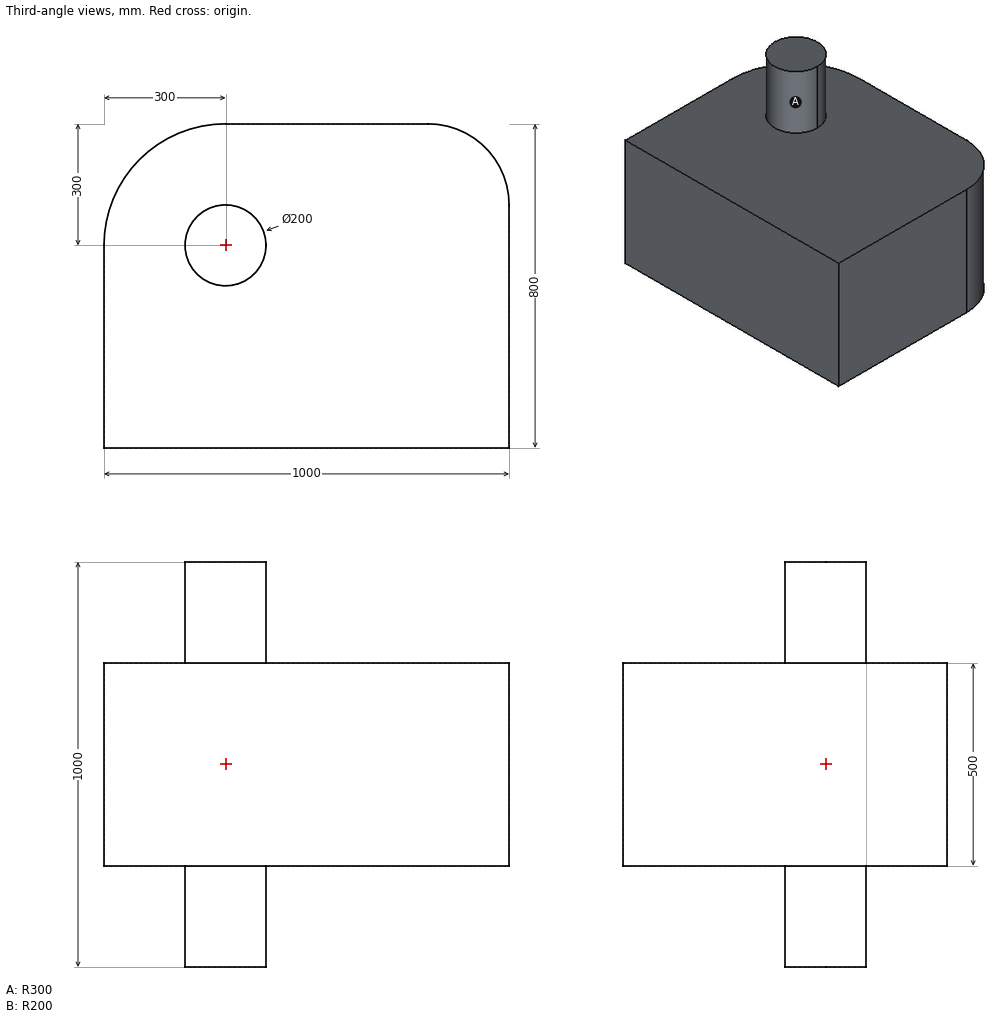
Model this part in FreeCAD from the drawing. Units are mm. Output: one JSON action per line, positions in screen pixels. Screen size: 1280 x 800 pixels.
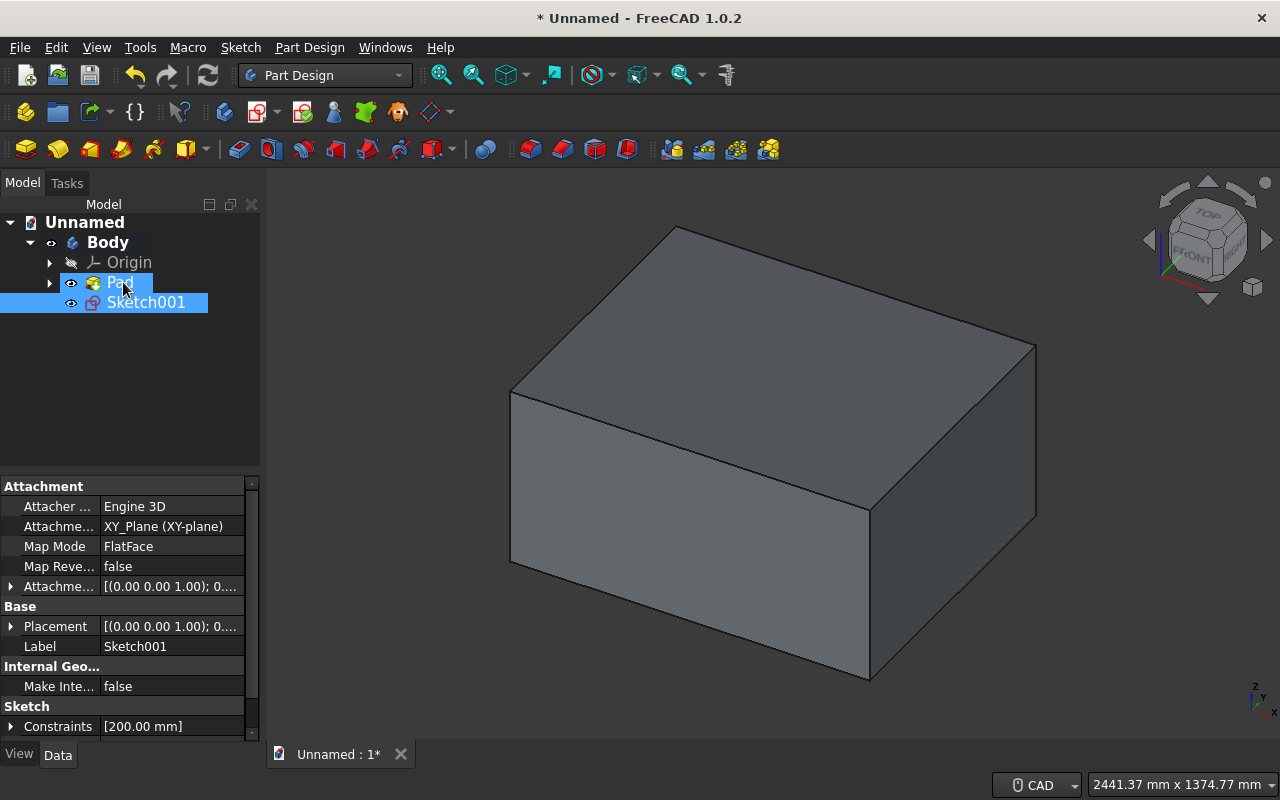
{"action": "left_click", "coordinate": [26, 150]}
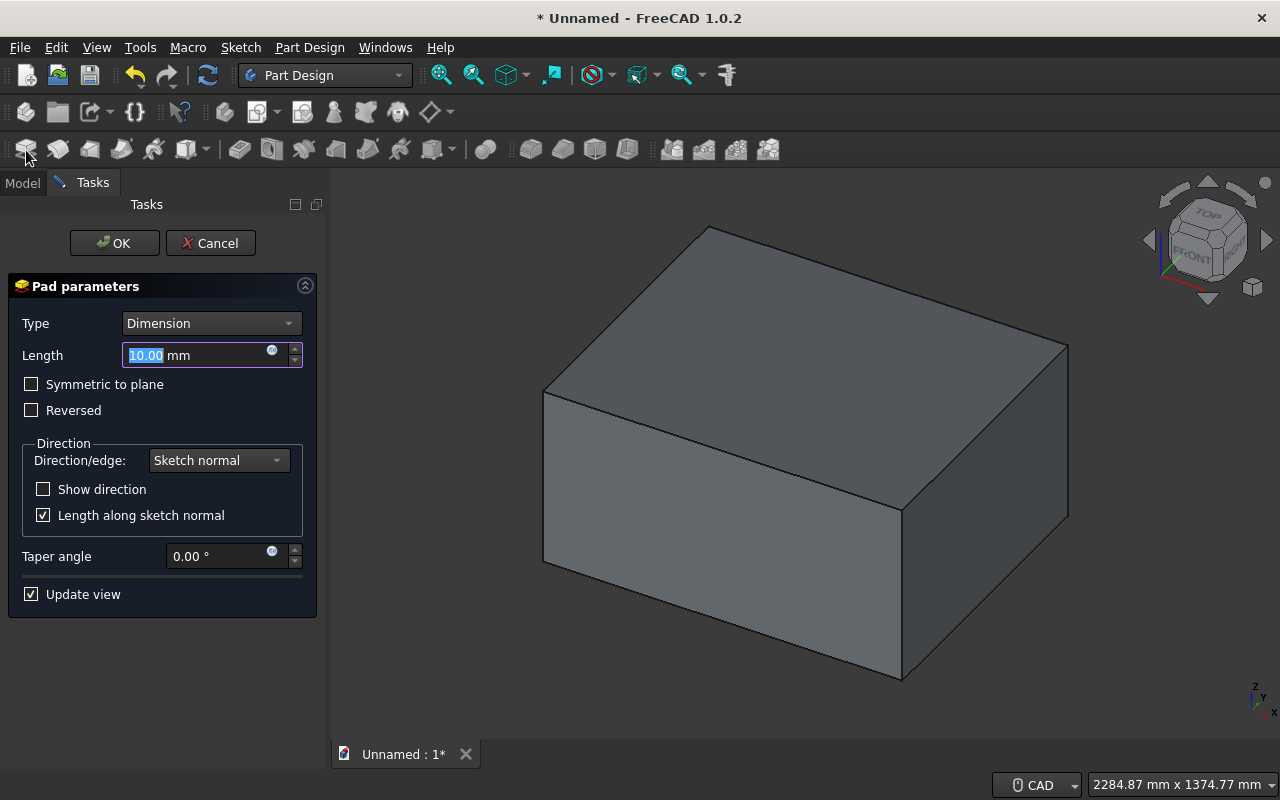
{"action": "type", "text": "1000"}
{"action": "key", "text": "Tab"}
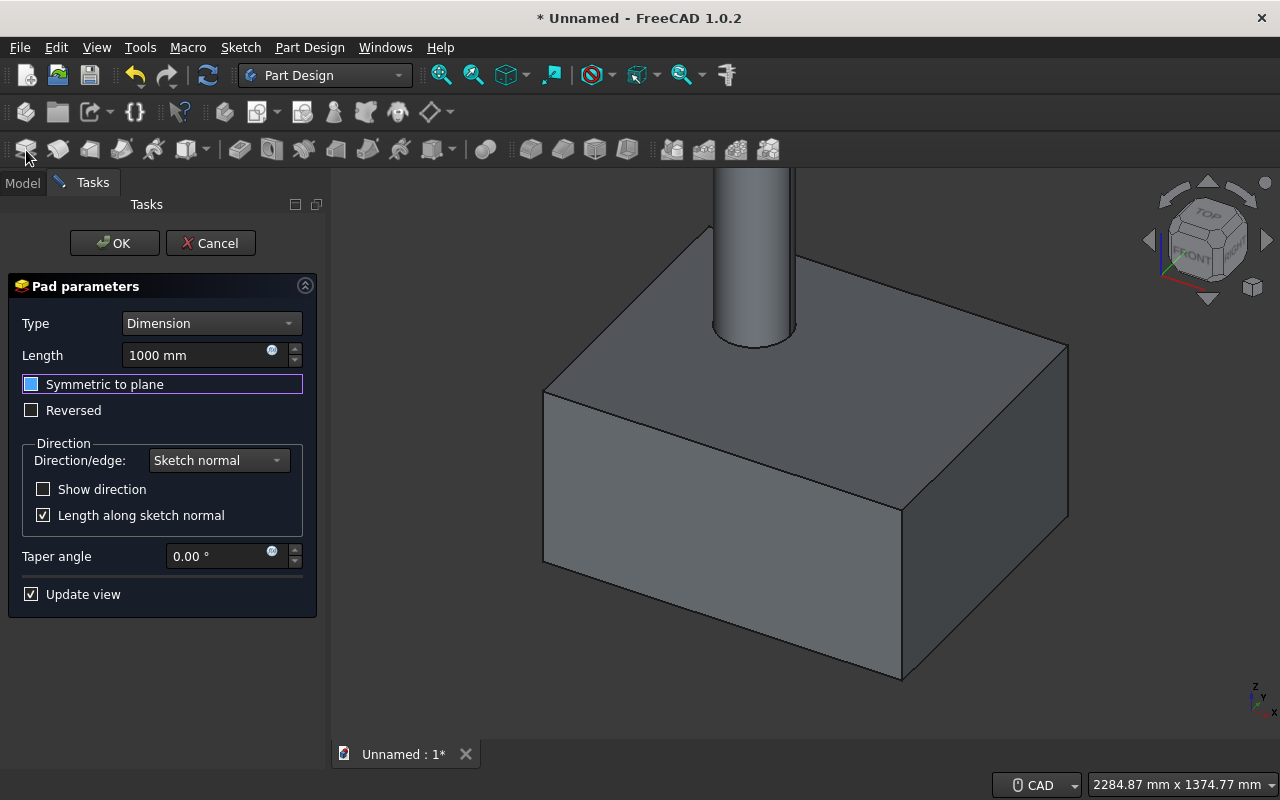
{"action": "left_click", "coordinate": [30, 384]}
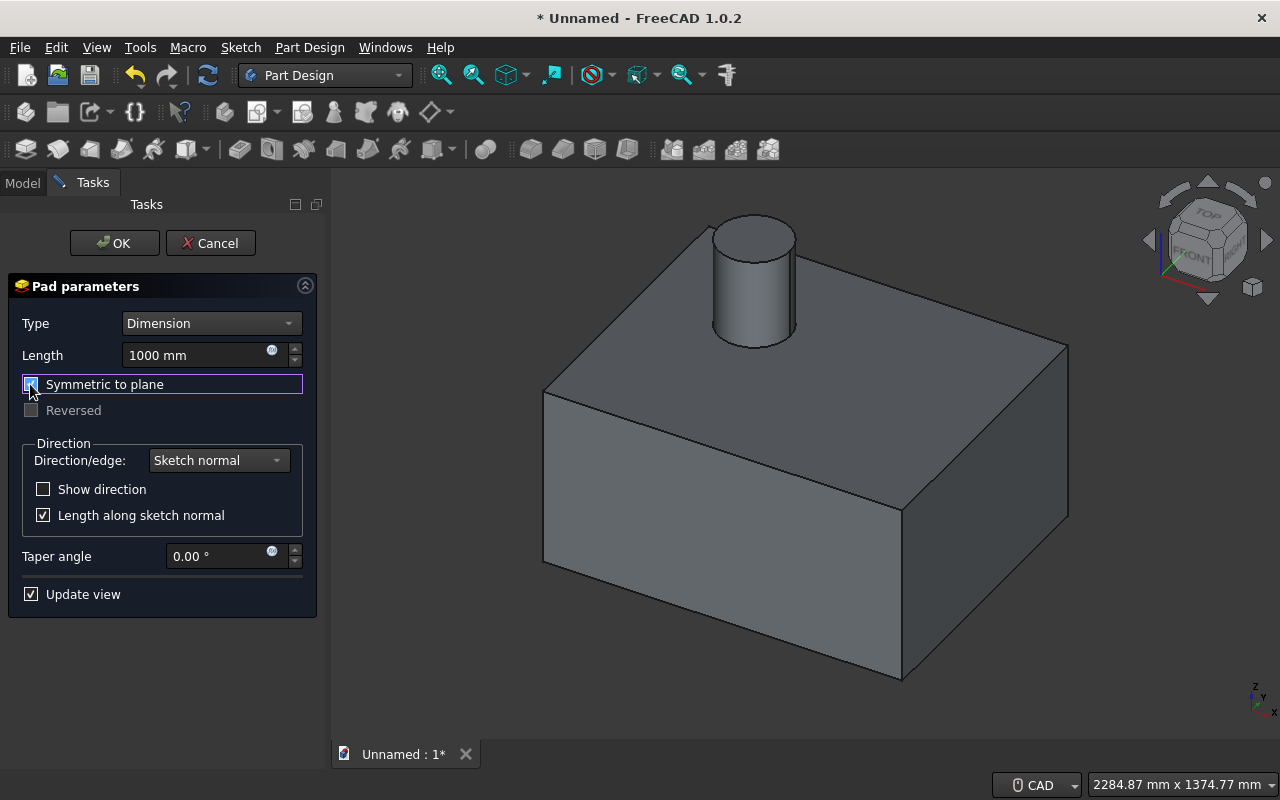
{"action": "left_click", "coordinate": [115, 243]}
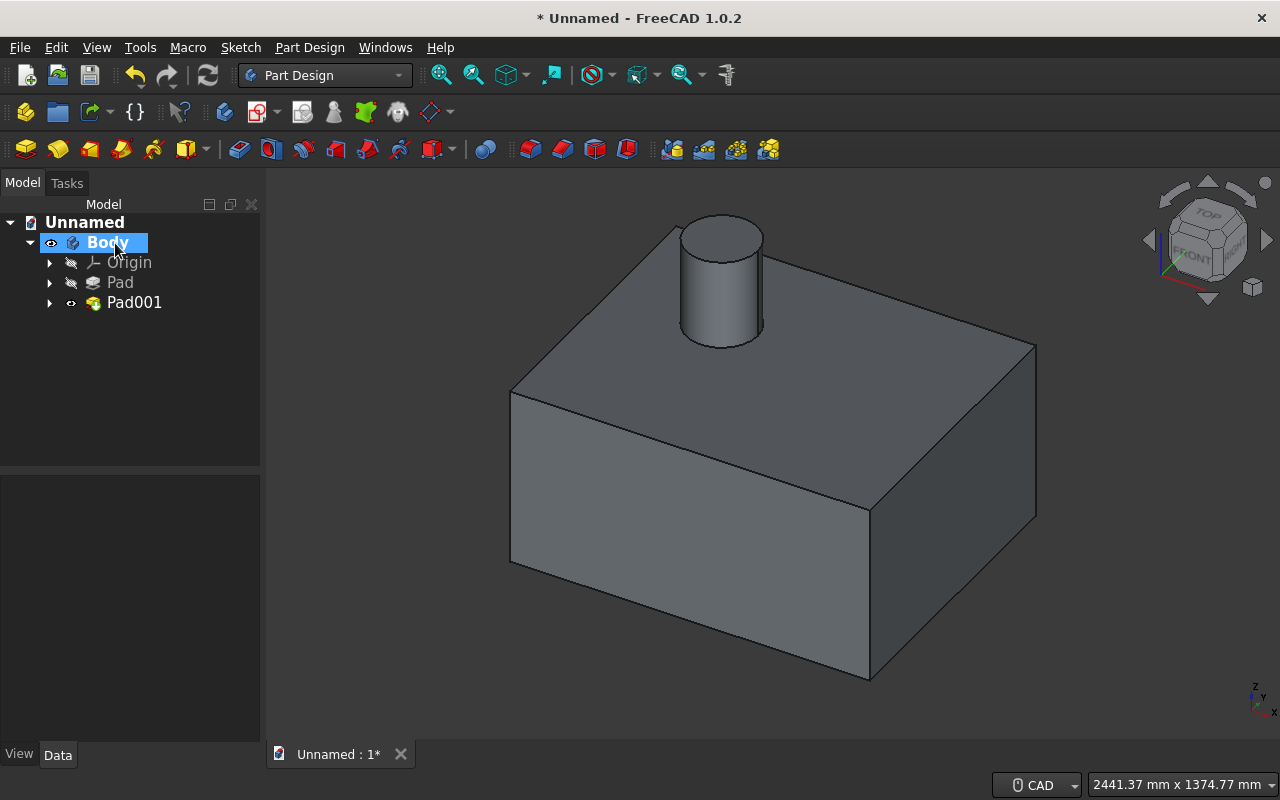
{"action": "key", "text": "v f"}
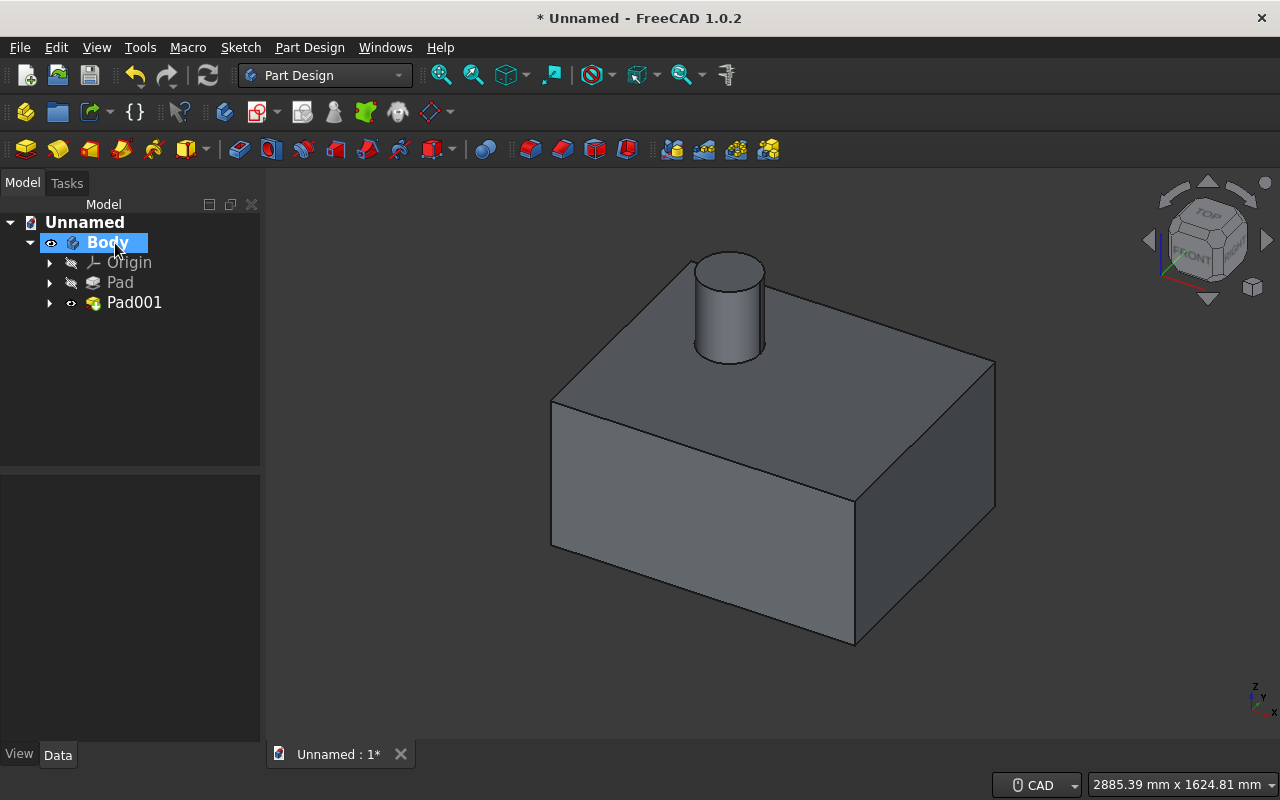
{"action": "key", "text": "0"}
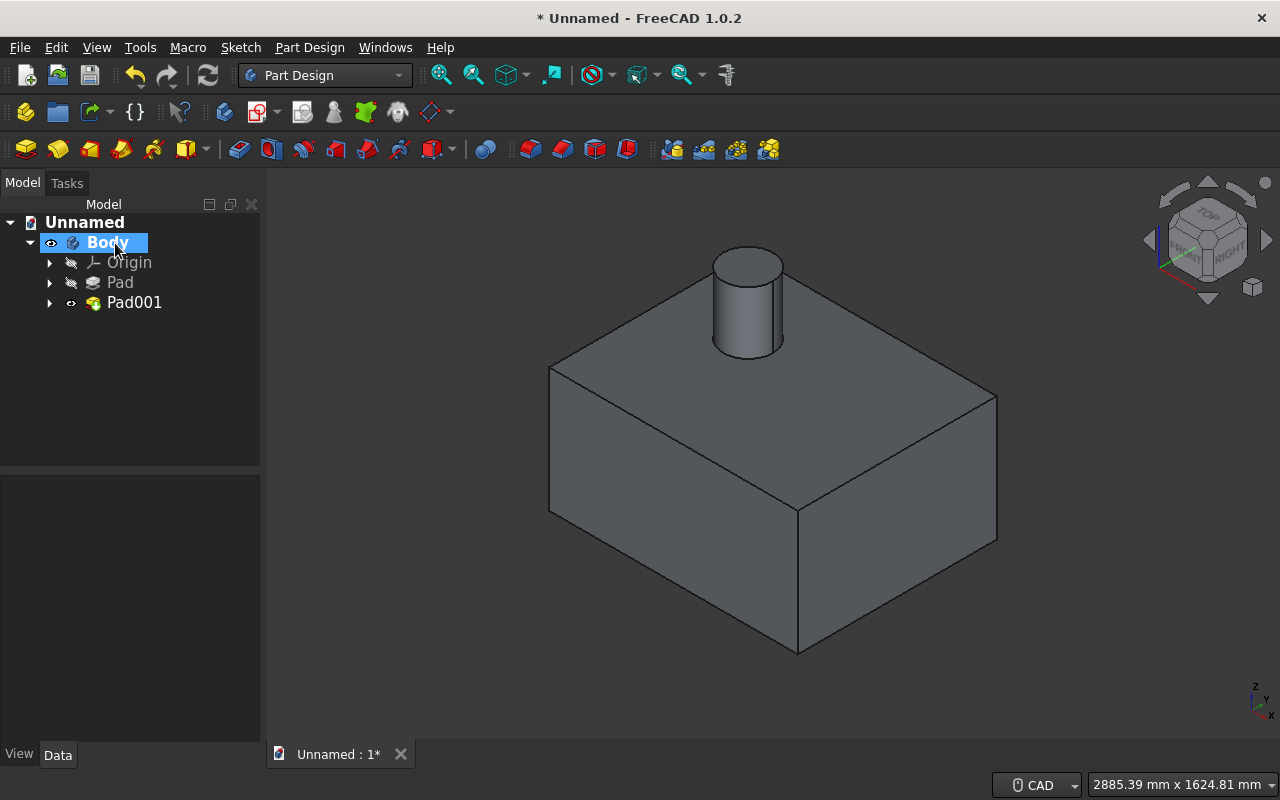
{"action": "key", "text": "2"}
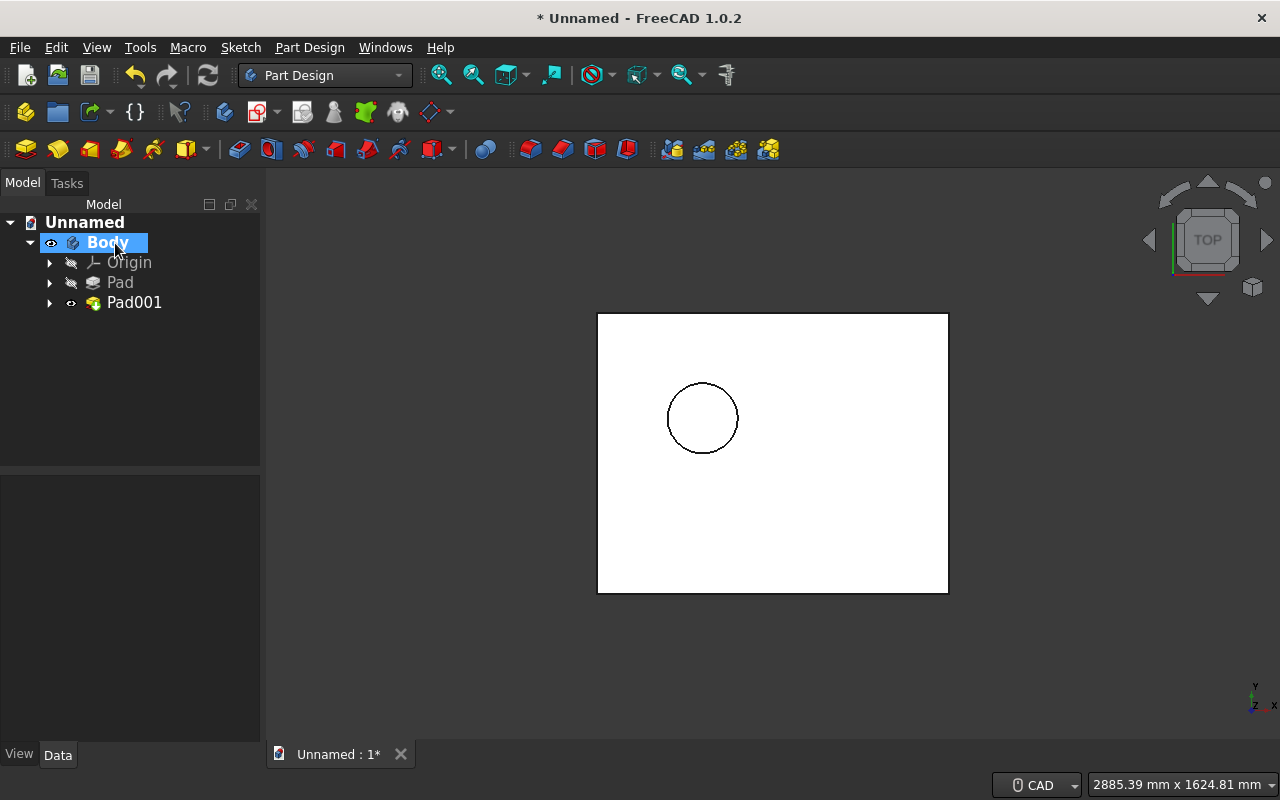
{"action": "key", "text": "1"}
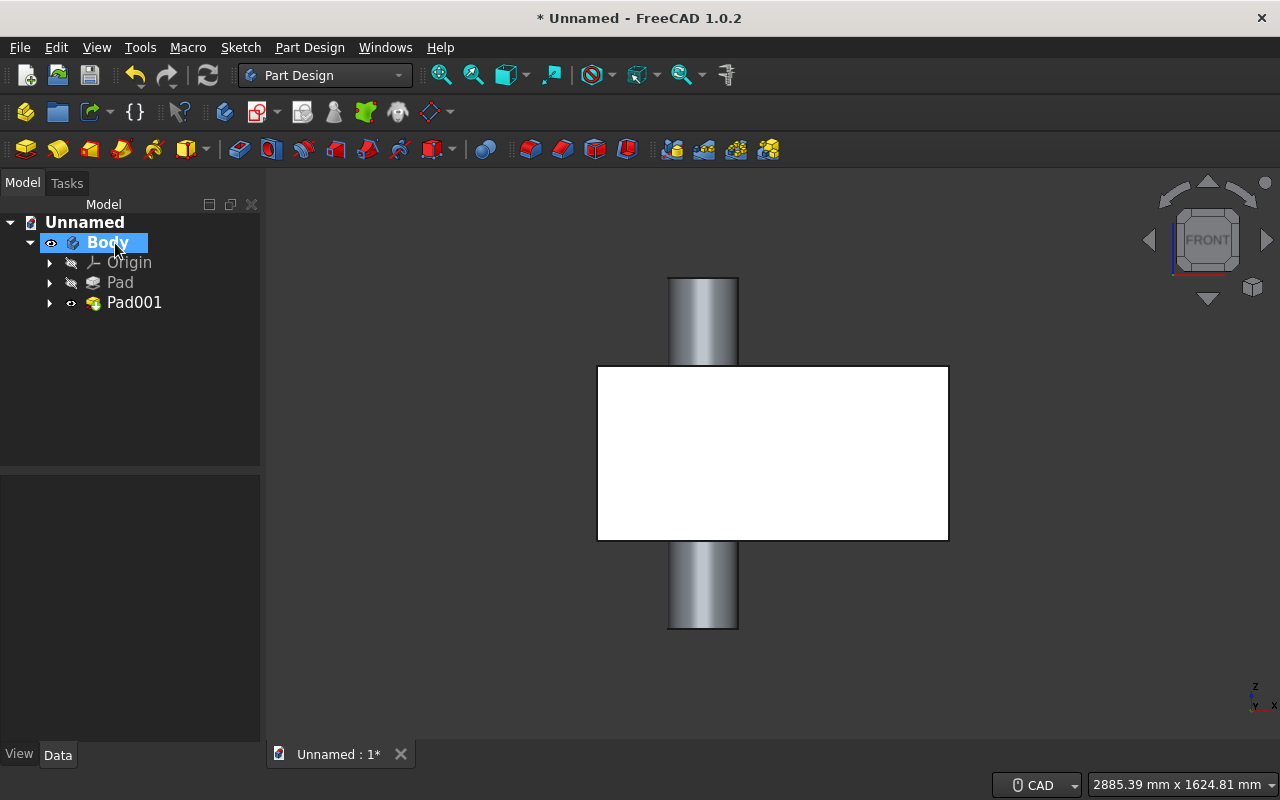
{"action": "key", "text": "3"}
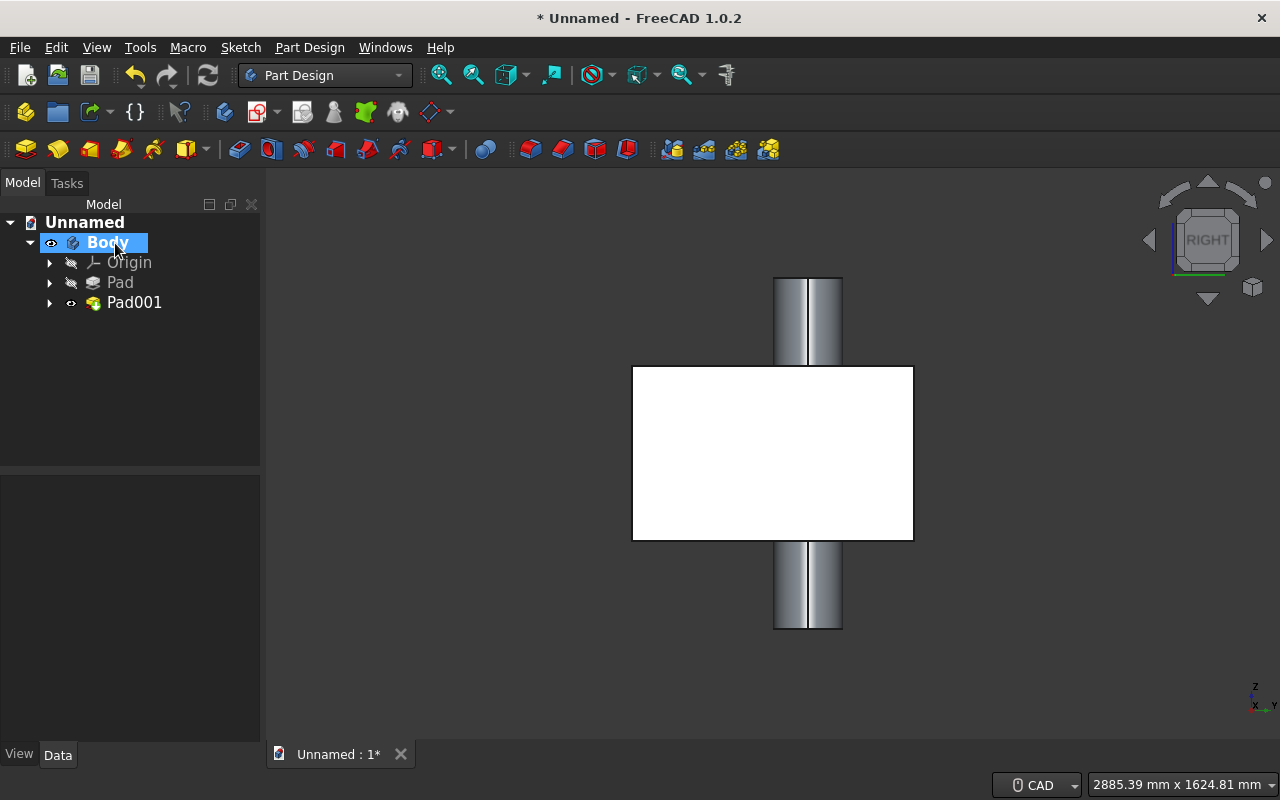
{"action": "key", "text": "5"}